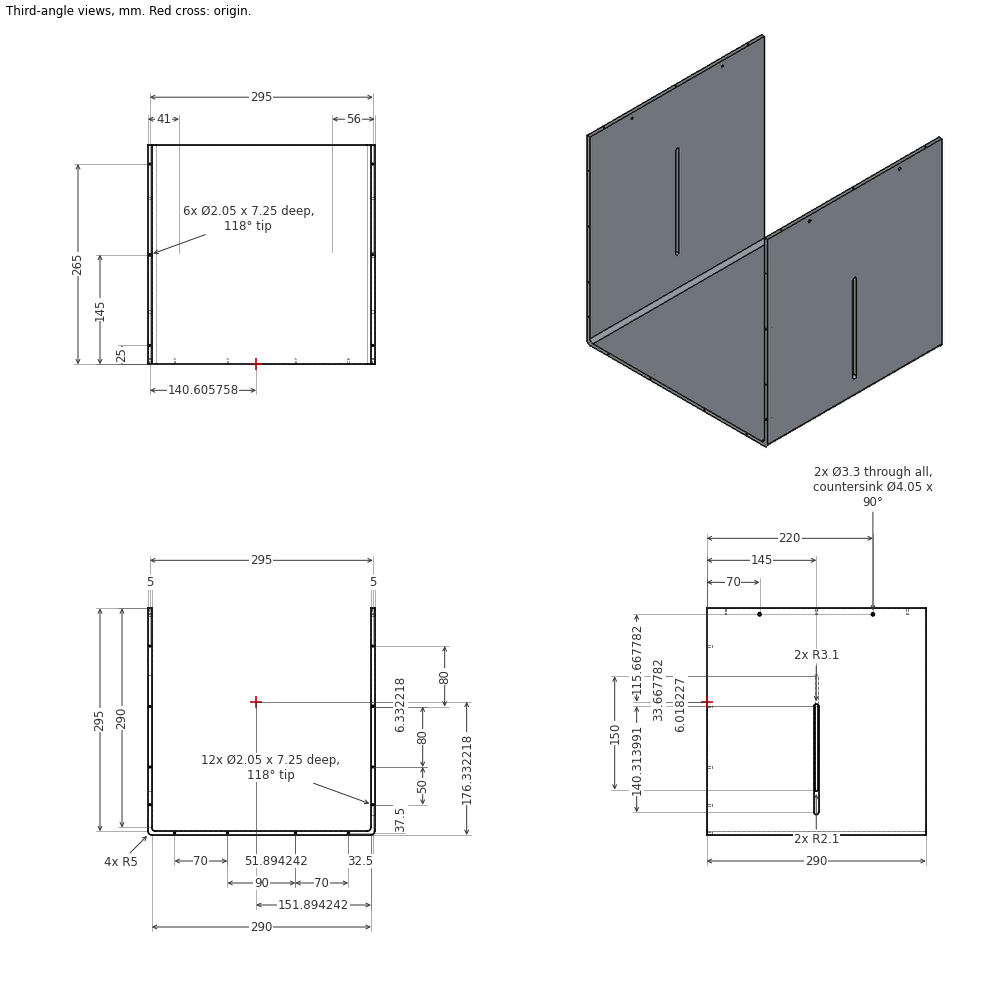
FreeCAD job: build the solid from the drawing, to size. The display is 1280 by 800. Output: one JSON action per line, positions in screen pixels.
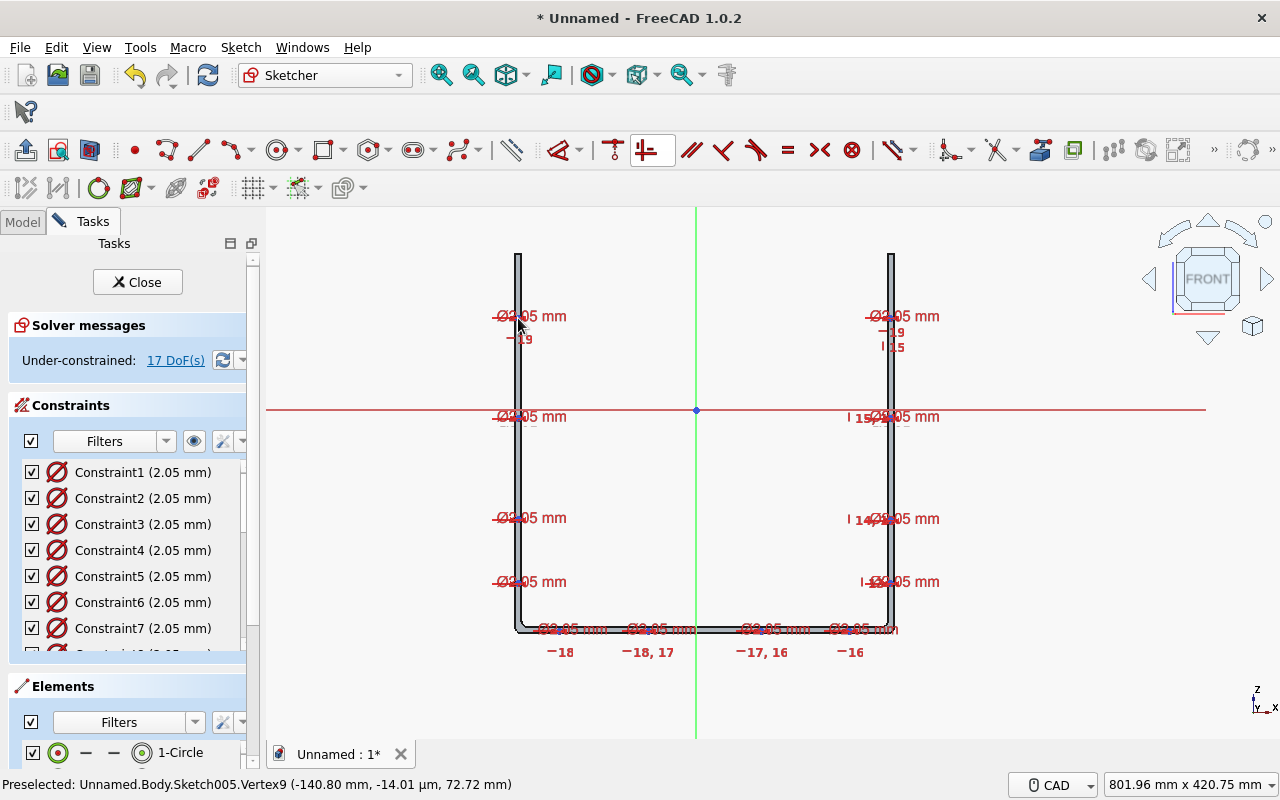
{"action": "left_click", "coordinate": [518, 318]}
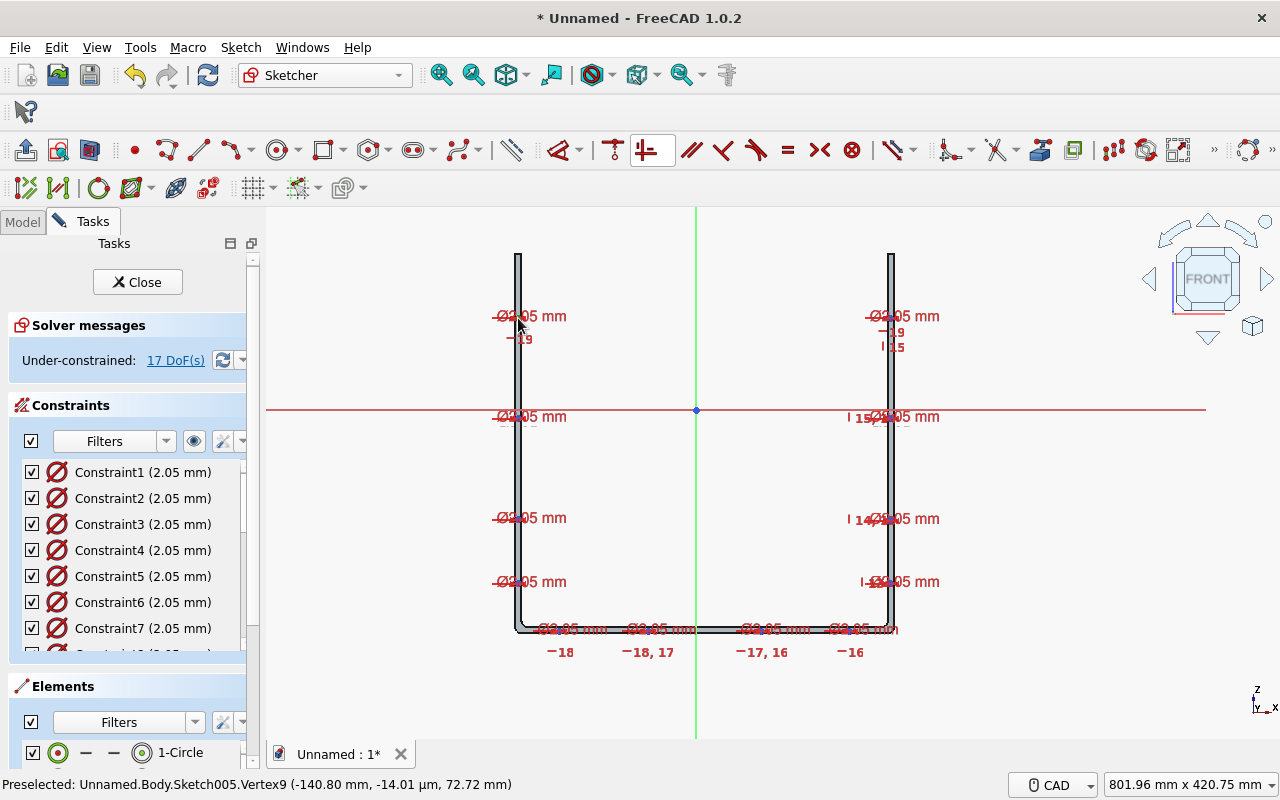
{"action": "left_click", "coordinate": [518, 419]}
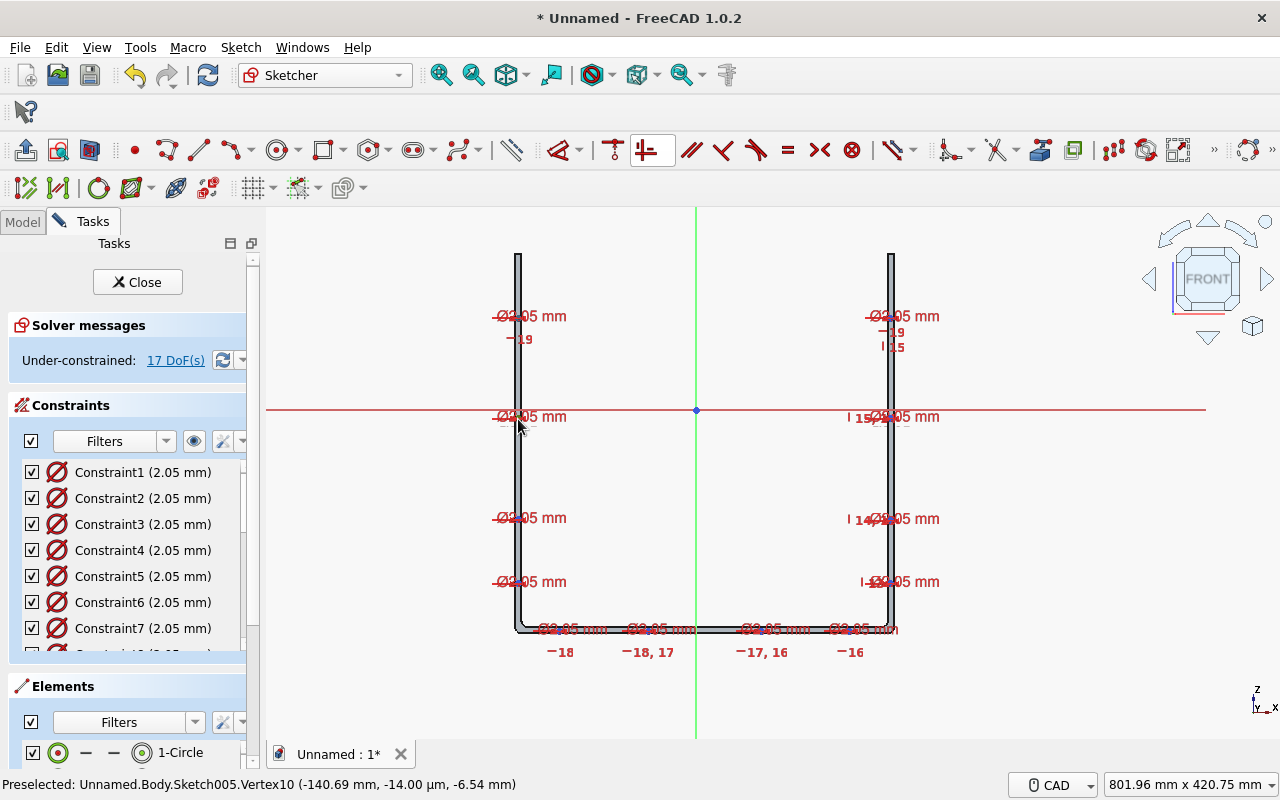
{"action": "key", "text": "v"}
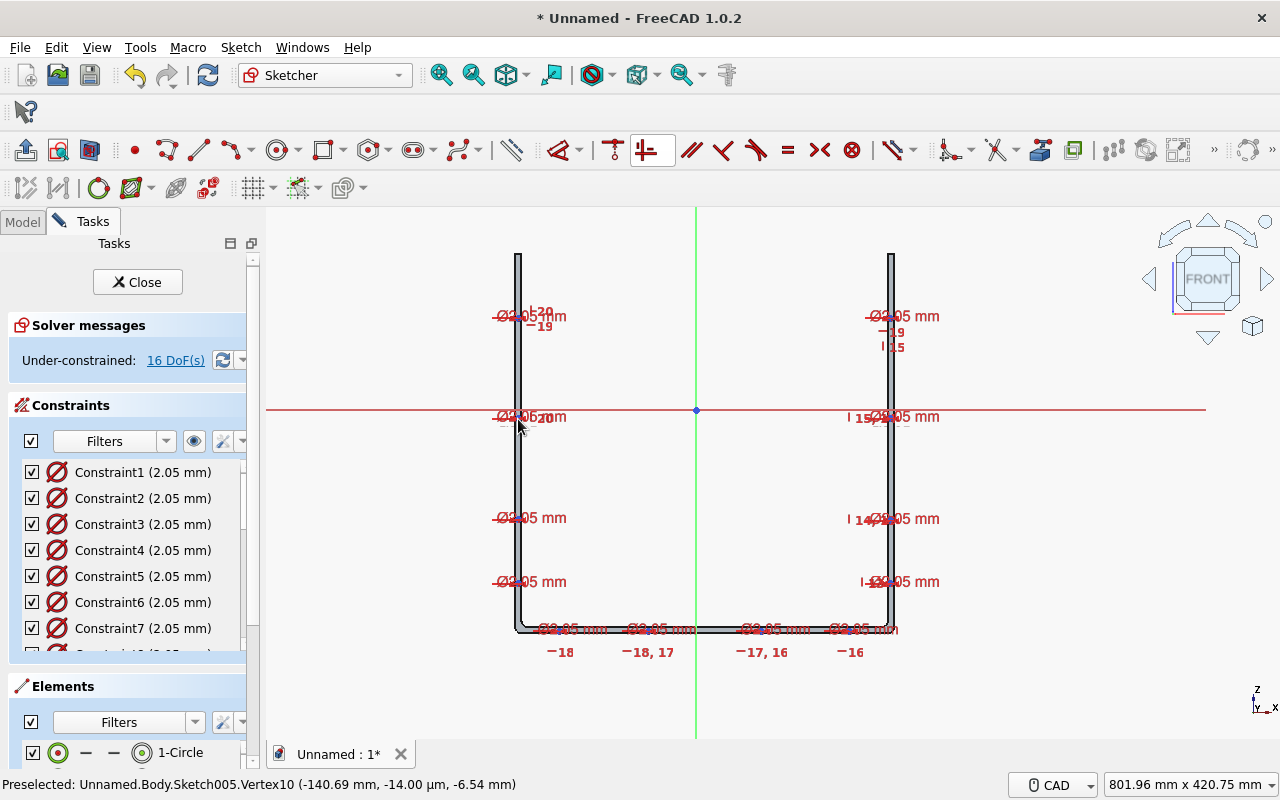
{"action": "left_click", "coordinate": [891, 419]}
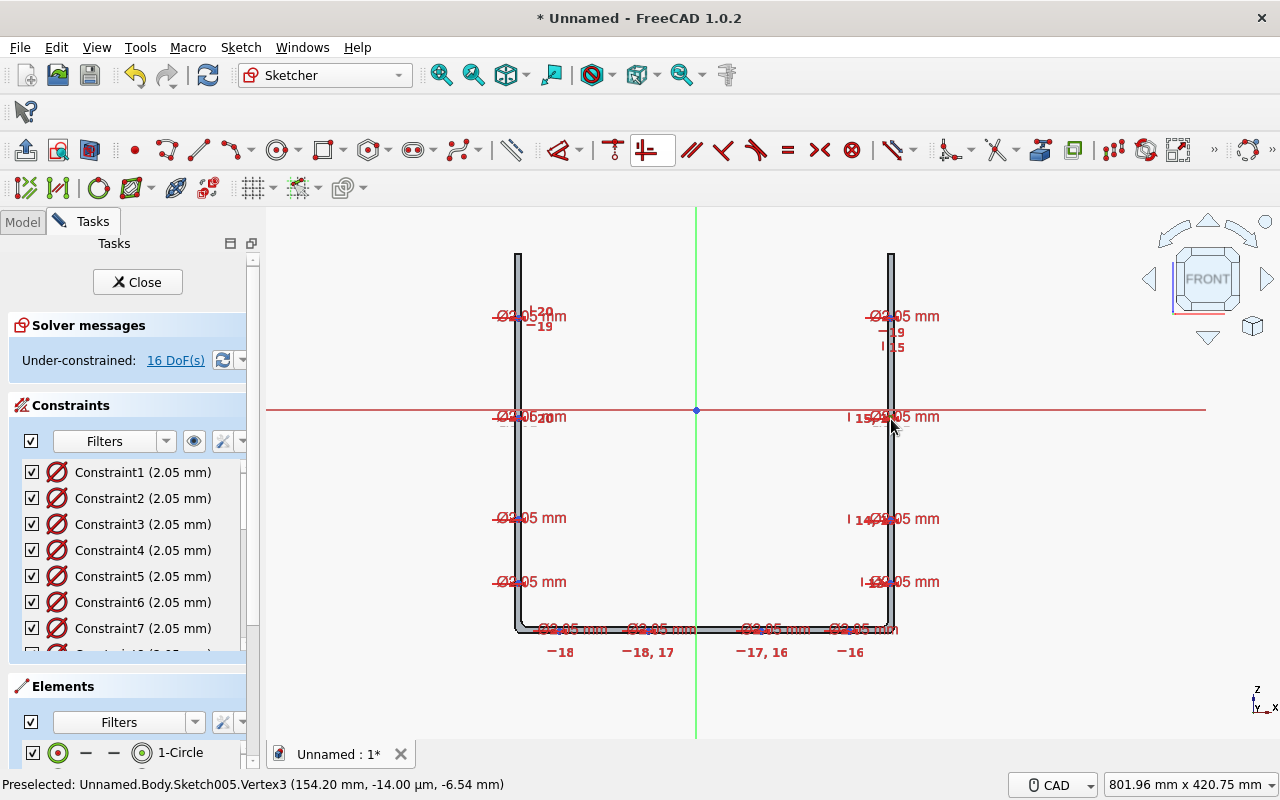
{"action": "left_click", "coordinate": [518, 419]}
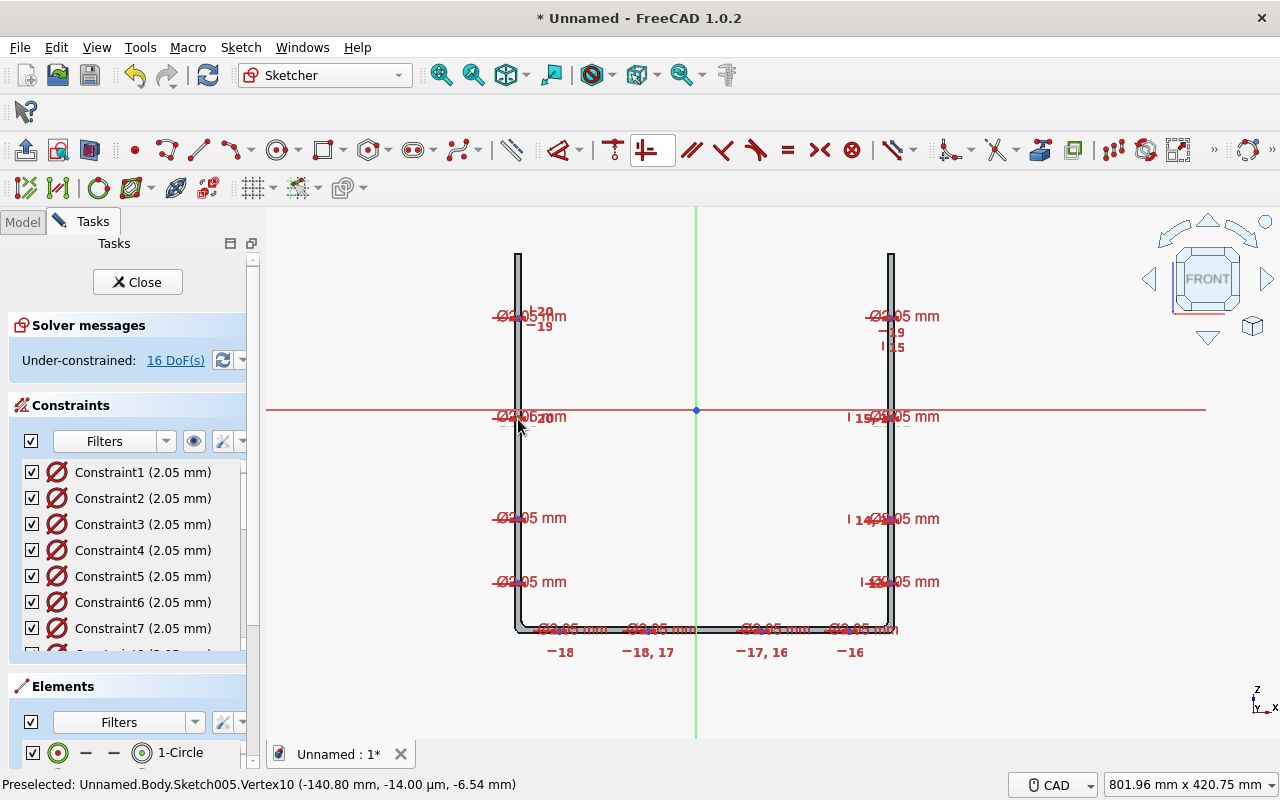
{"action": "left_click", "coordinate": [670, 150]}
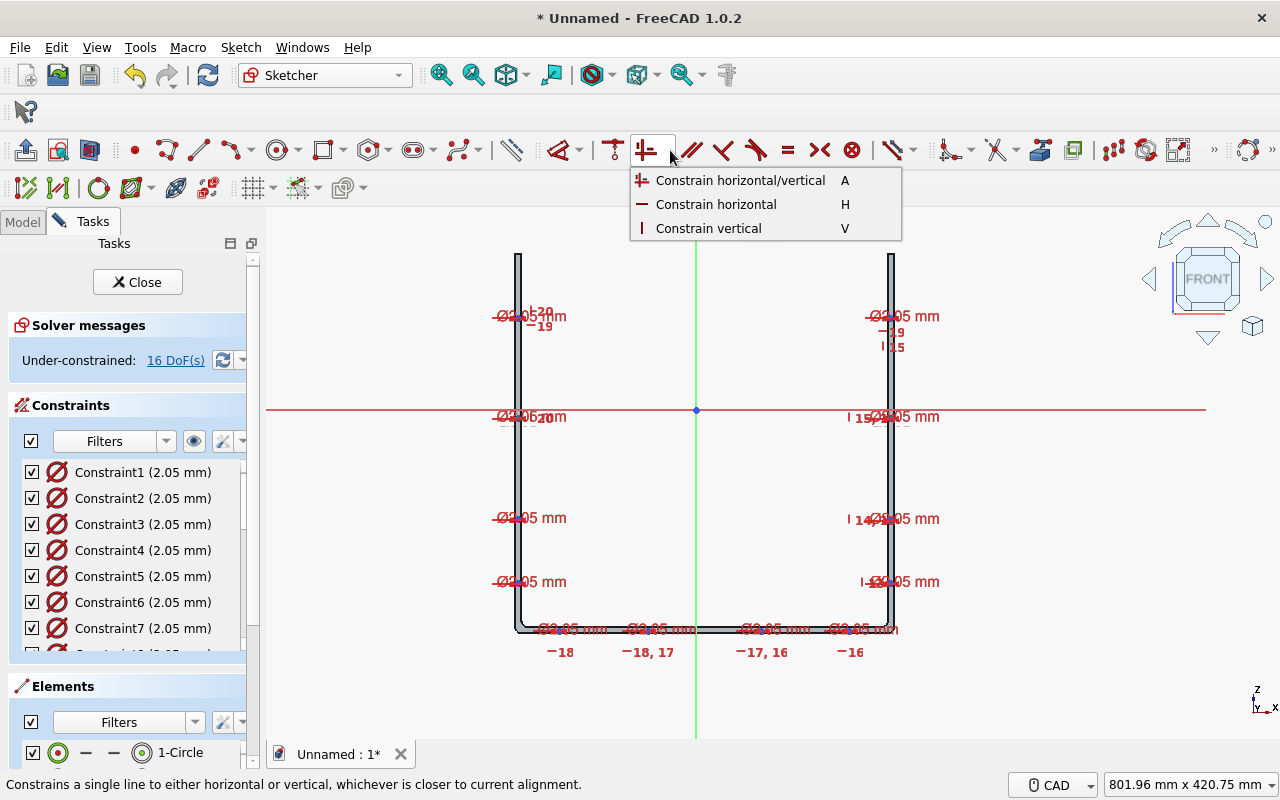
{"action": "left_click", "coordinate": [766, 204]}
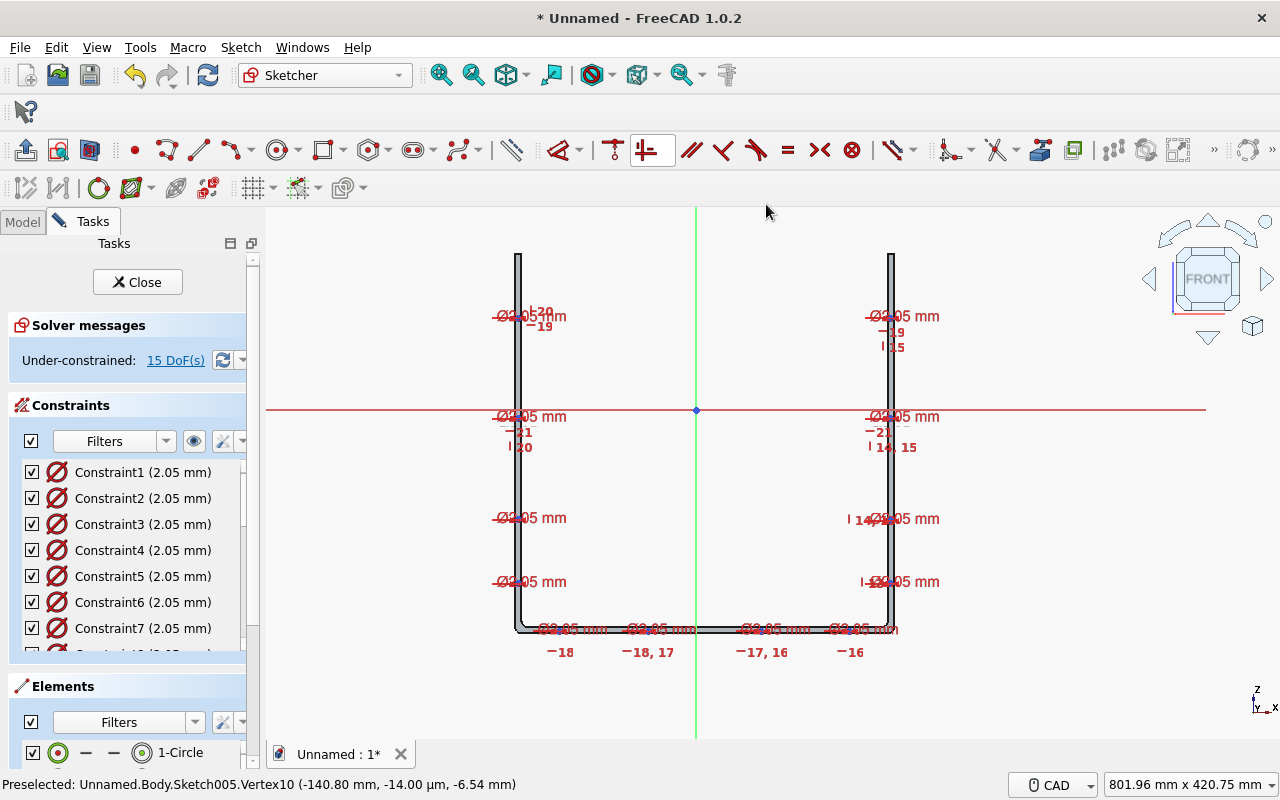
{"action": "left_click", "coordinate": [518, 419]}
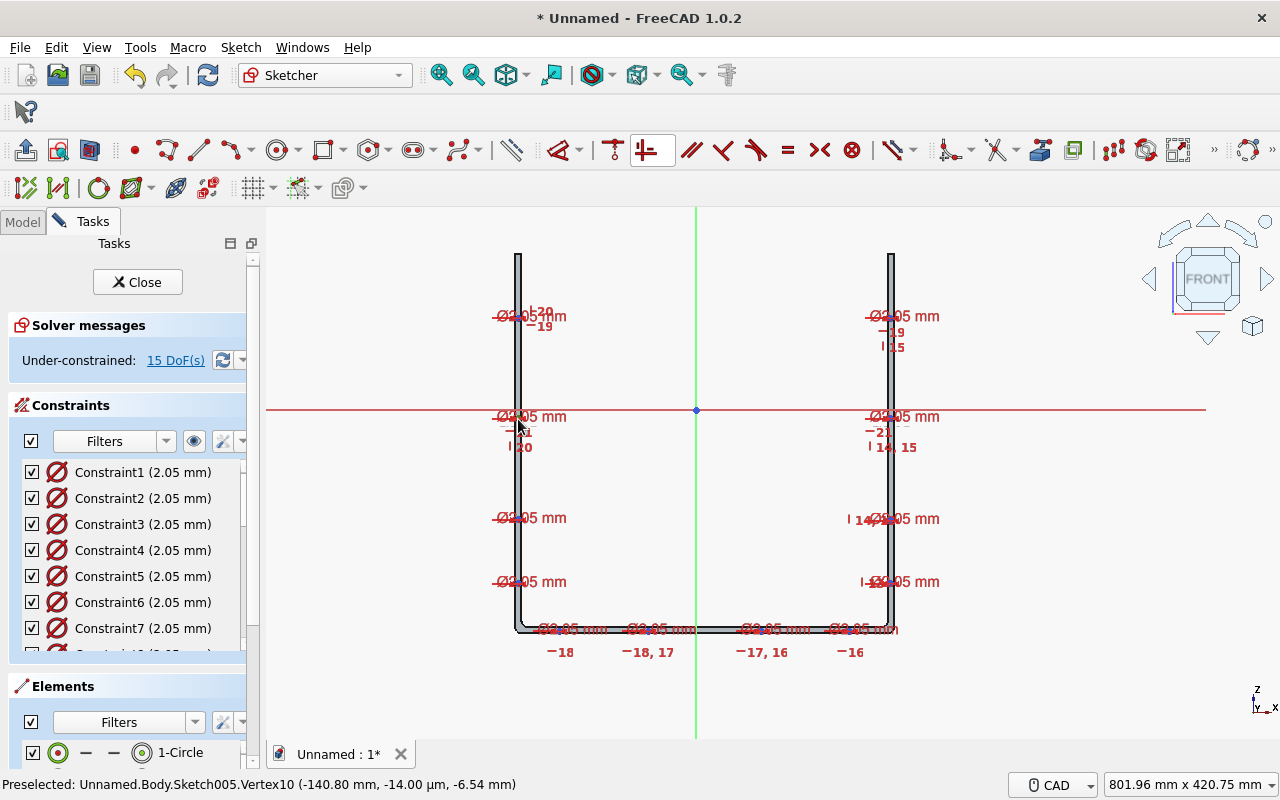
{"action": "left_click", "coordinate": [518, 520]}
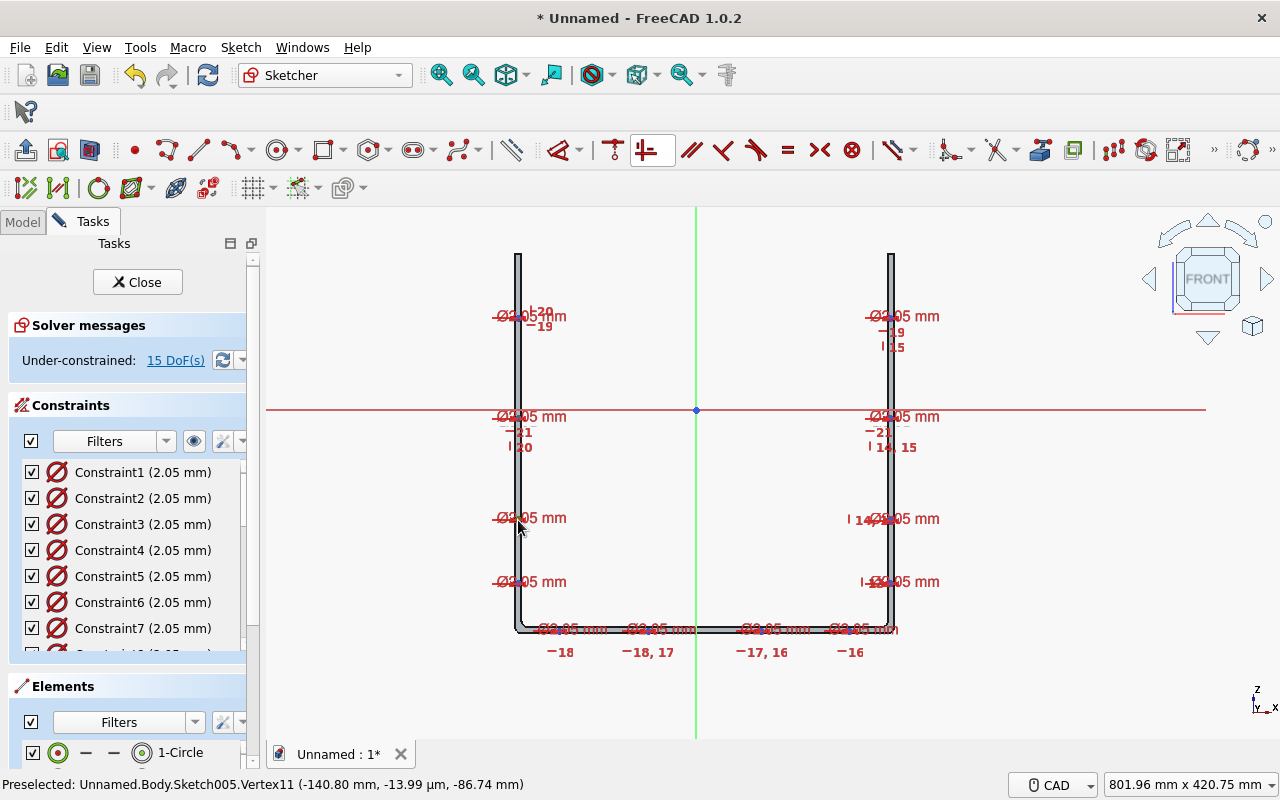
{"action": "key", "text": "v"}